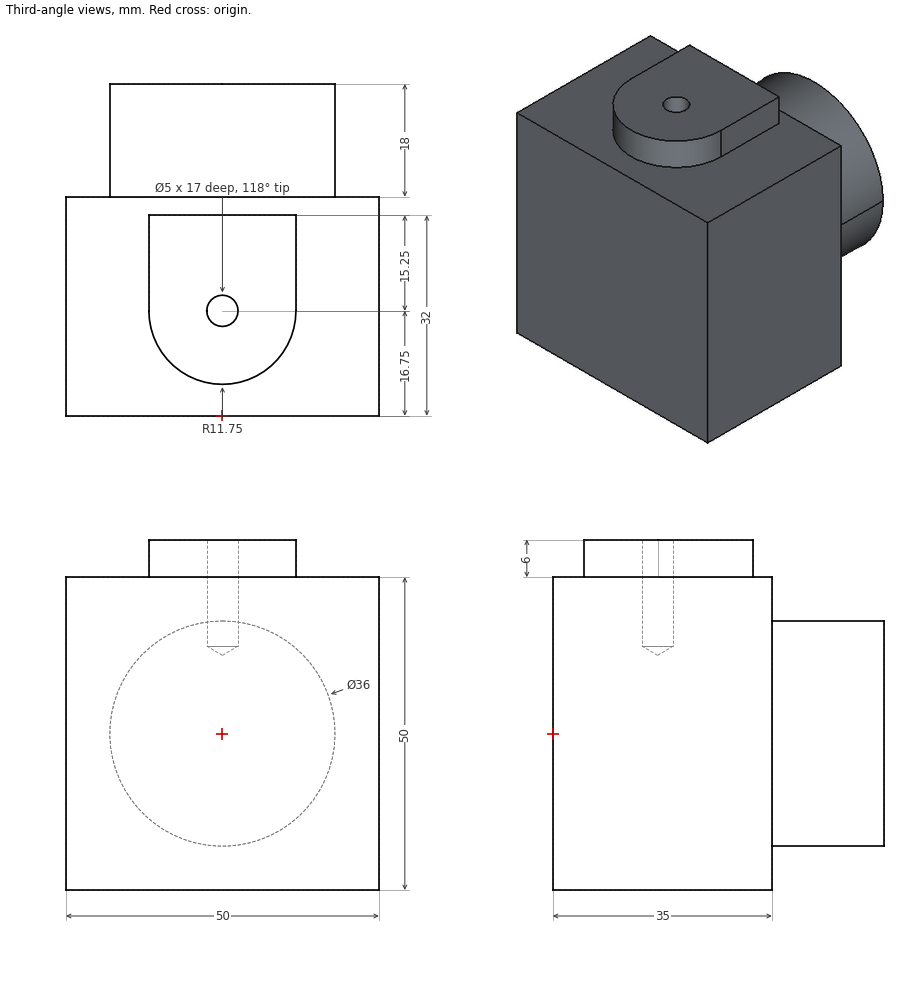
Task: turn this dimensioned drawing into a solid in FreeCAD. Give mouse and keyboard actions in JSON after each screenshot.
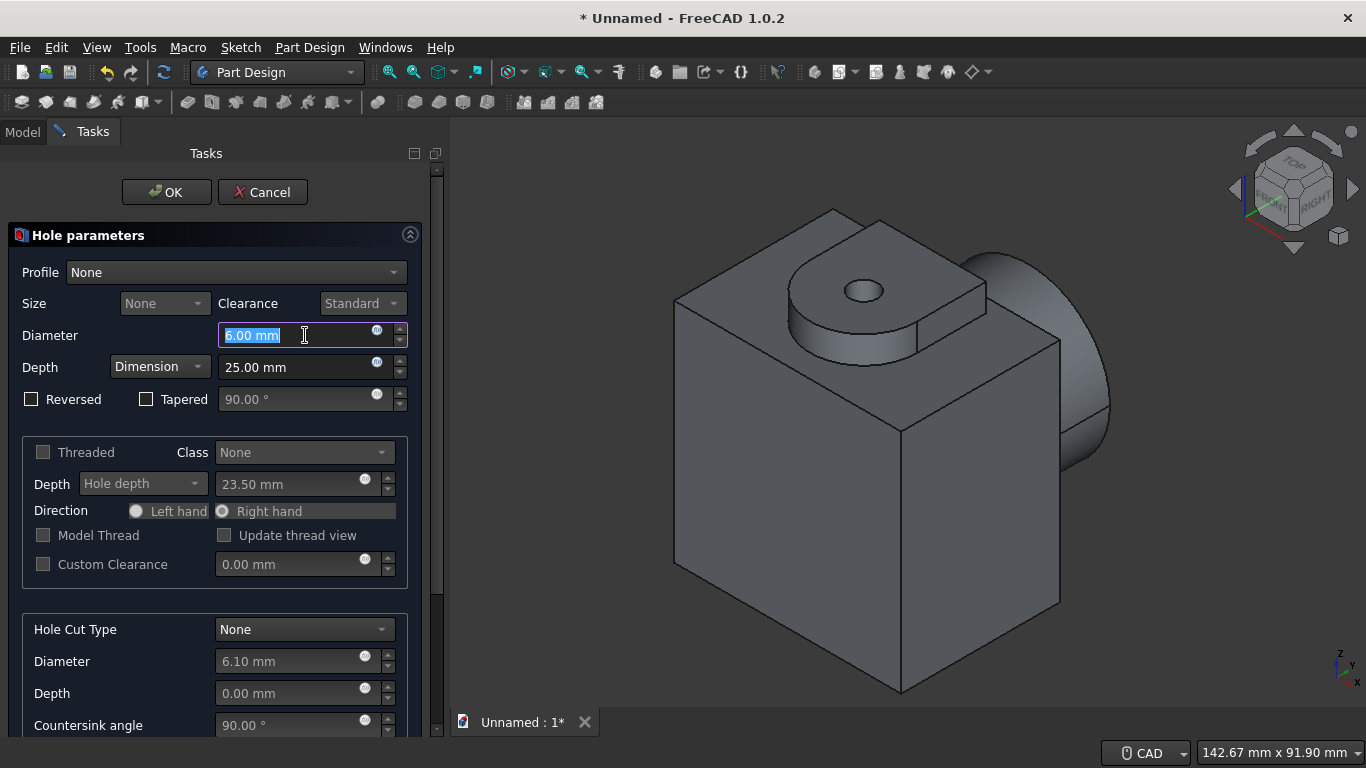
{"action": "type", "text": "5"}
{"action": "key", "text": "Tab"}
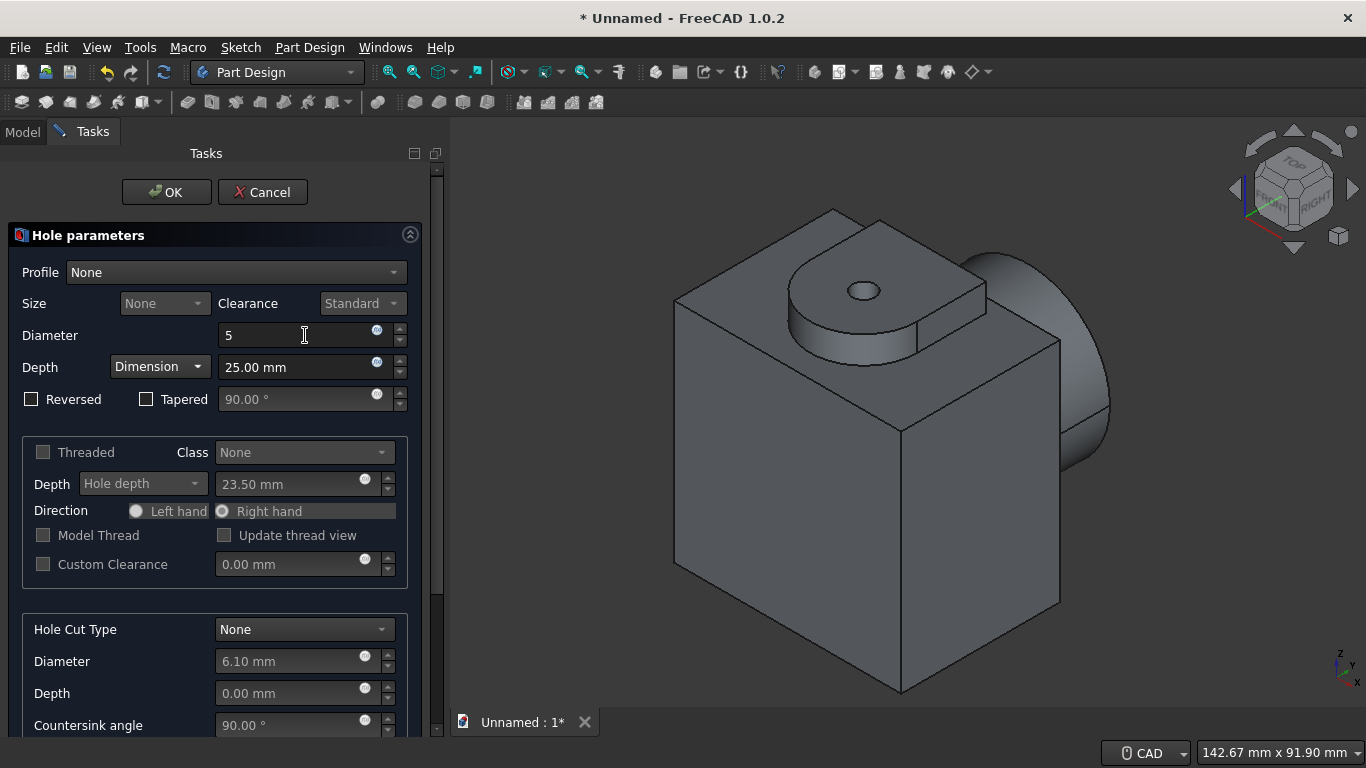
{"action": "triple_click", "coordinate": [305, 367]}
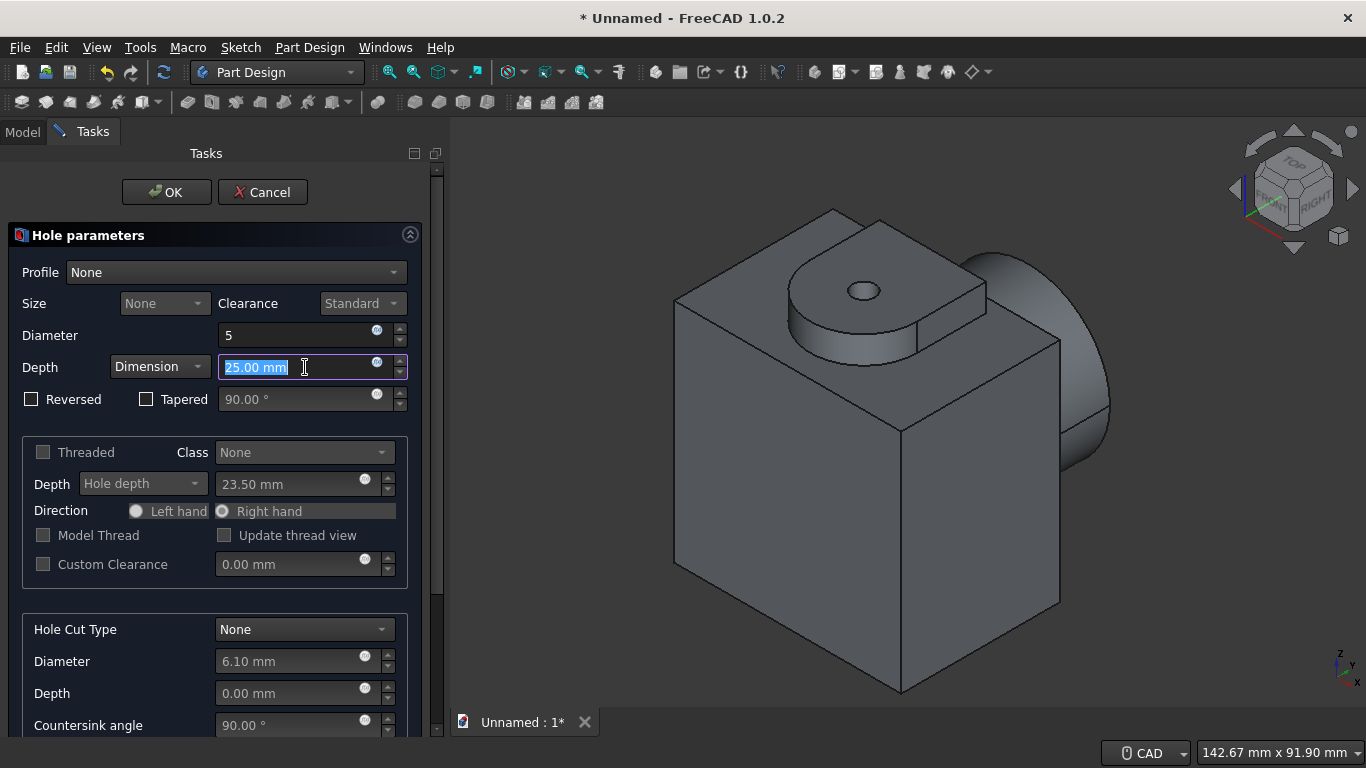
{"action": "type", "text": "17"}
{"action": "key", "text": "Tab"}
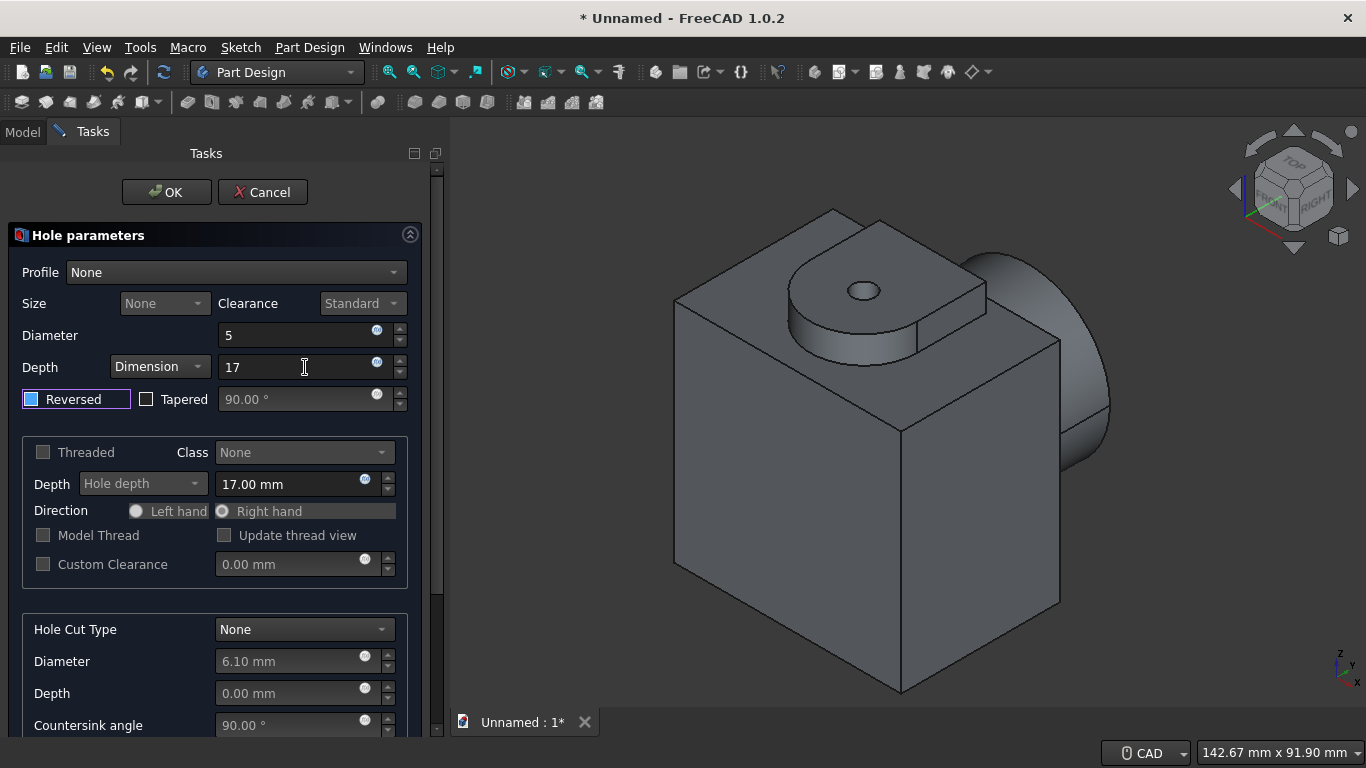
{"action": "left_click", "coordinate": [167, 192]}